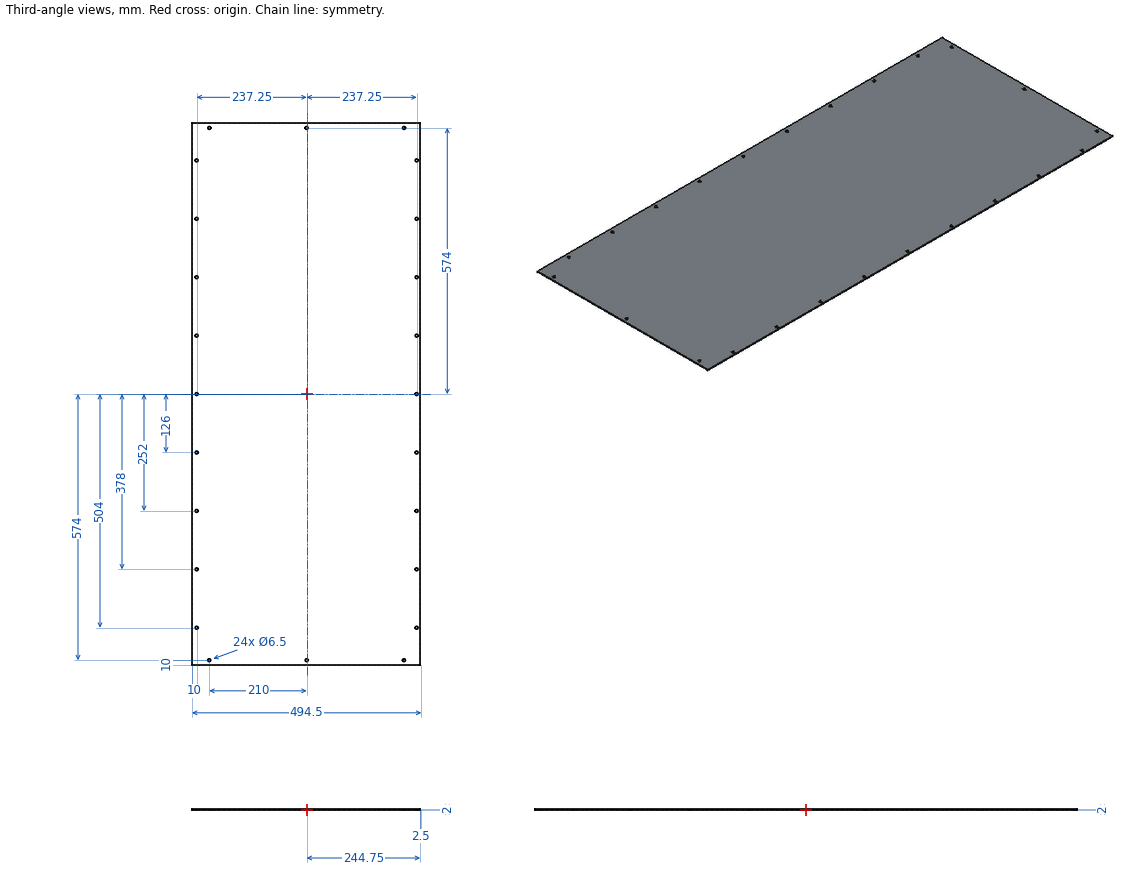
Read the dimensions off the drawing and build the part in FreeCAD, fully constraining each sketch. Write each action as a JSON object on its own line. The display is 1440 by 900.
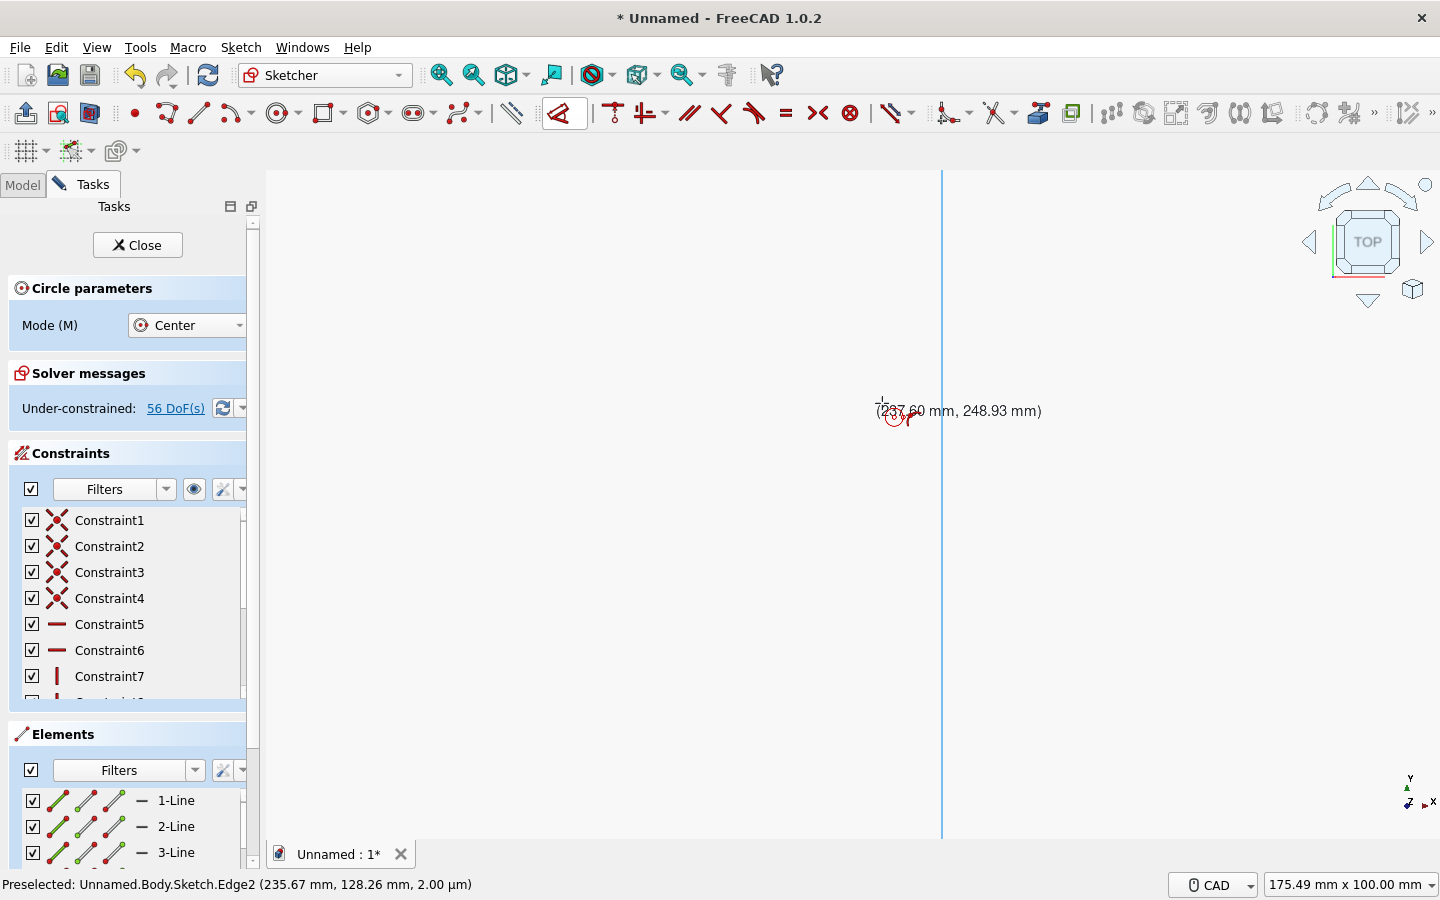
{"action": "scroll", "coordinate": [882, 403], "scroll_direction": "down", "scroll_amount": 15}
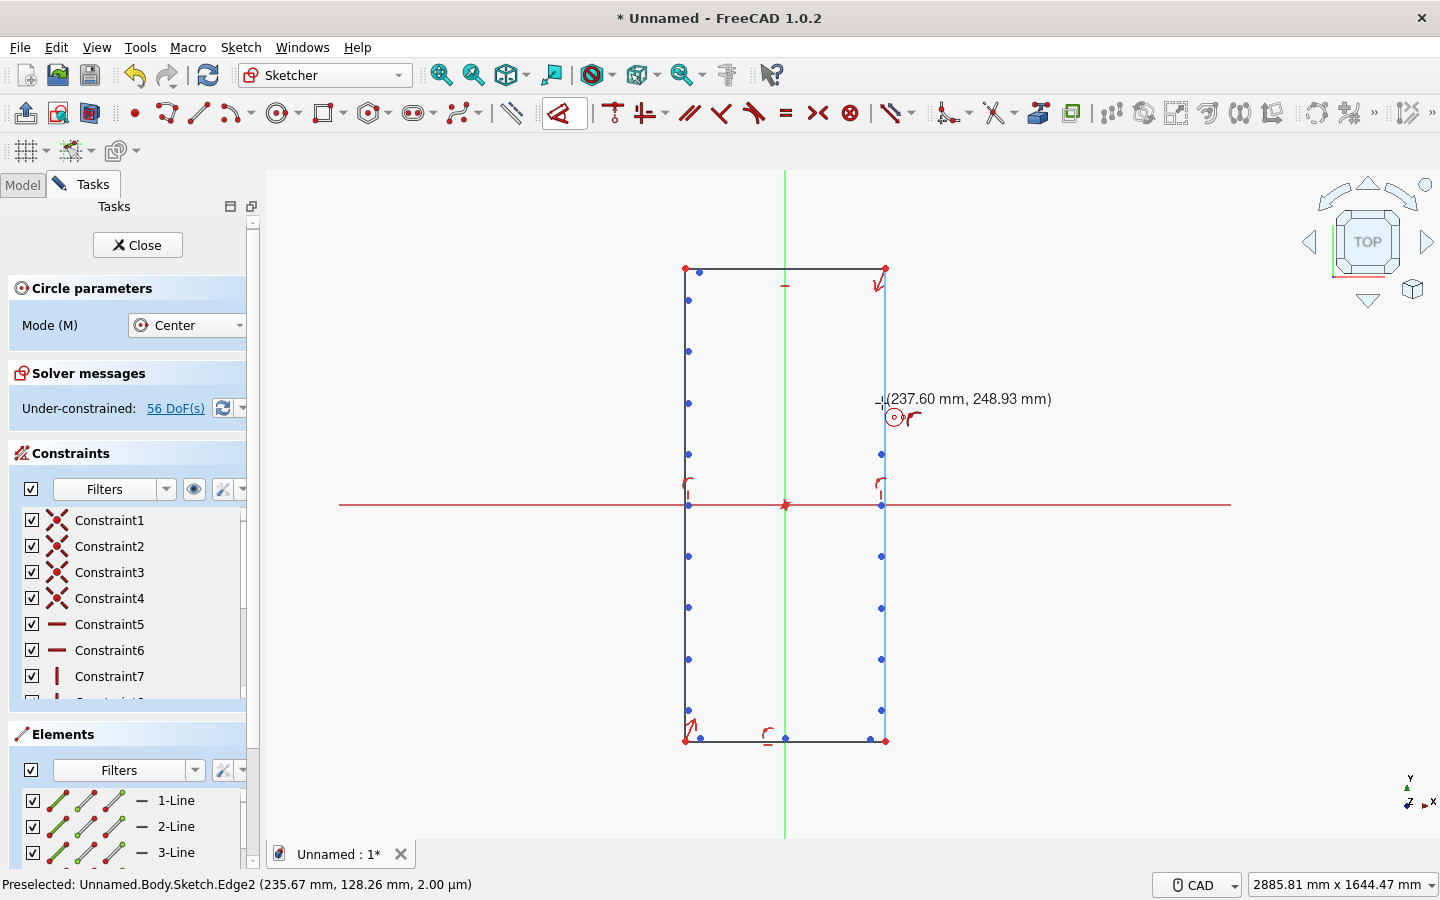
{"action": "scroll", "coordinate": [882, 403], "scroll_direction": "up", "scroll_amount": 7}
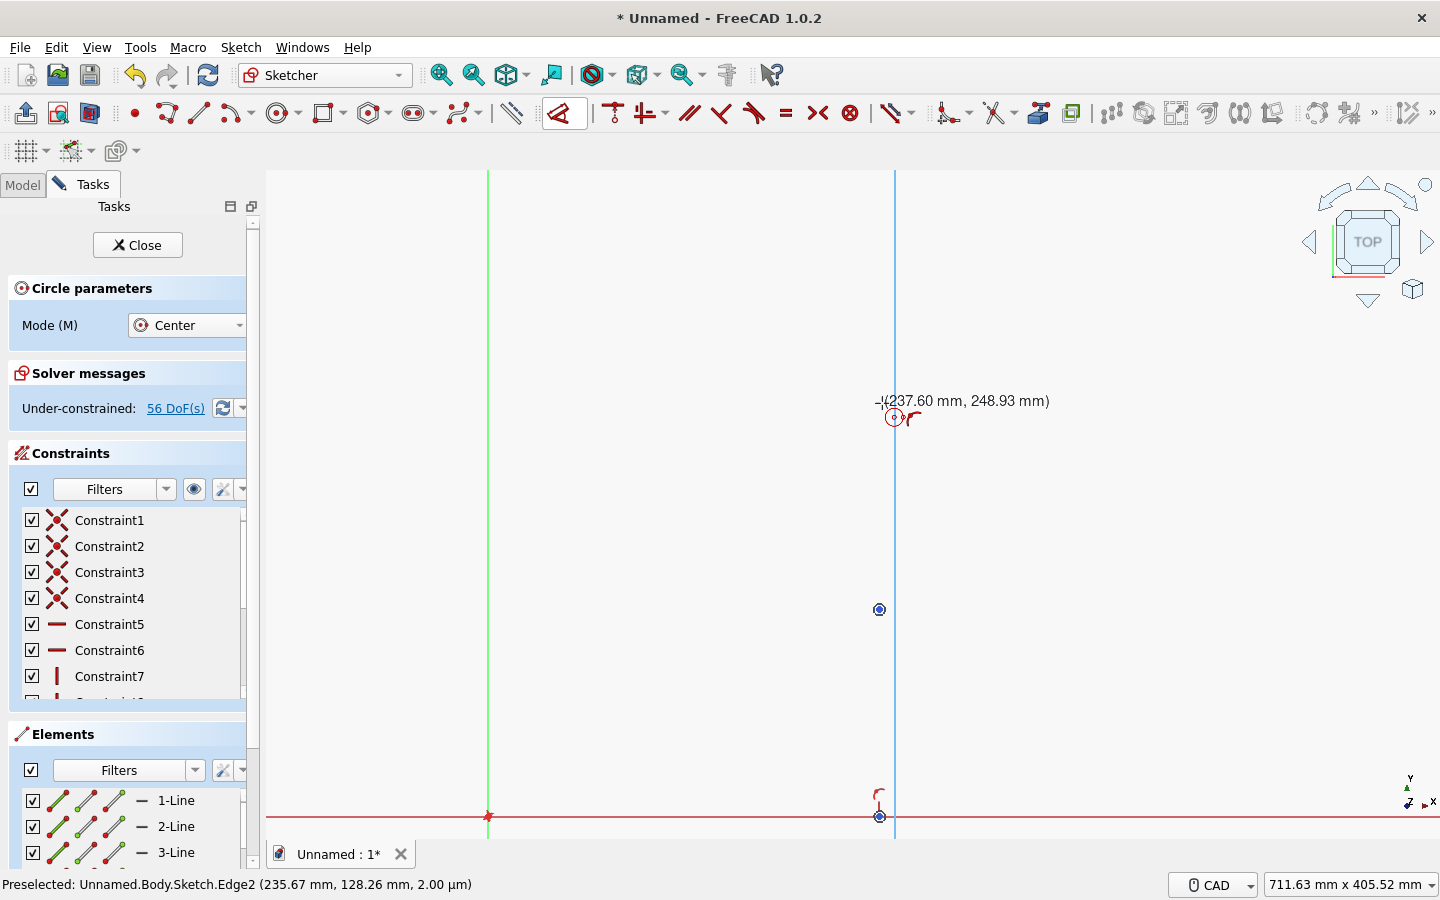
{"action": "left_click", "coordinate": [880, 401]}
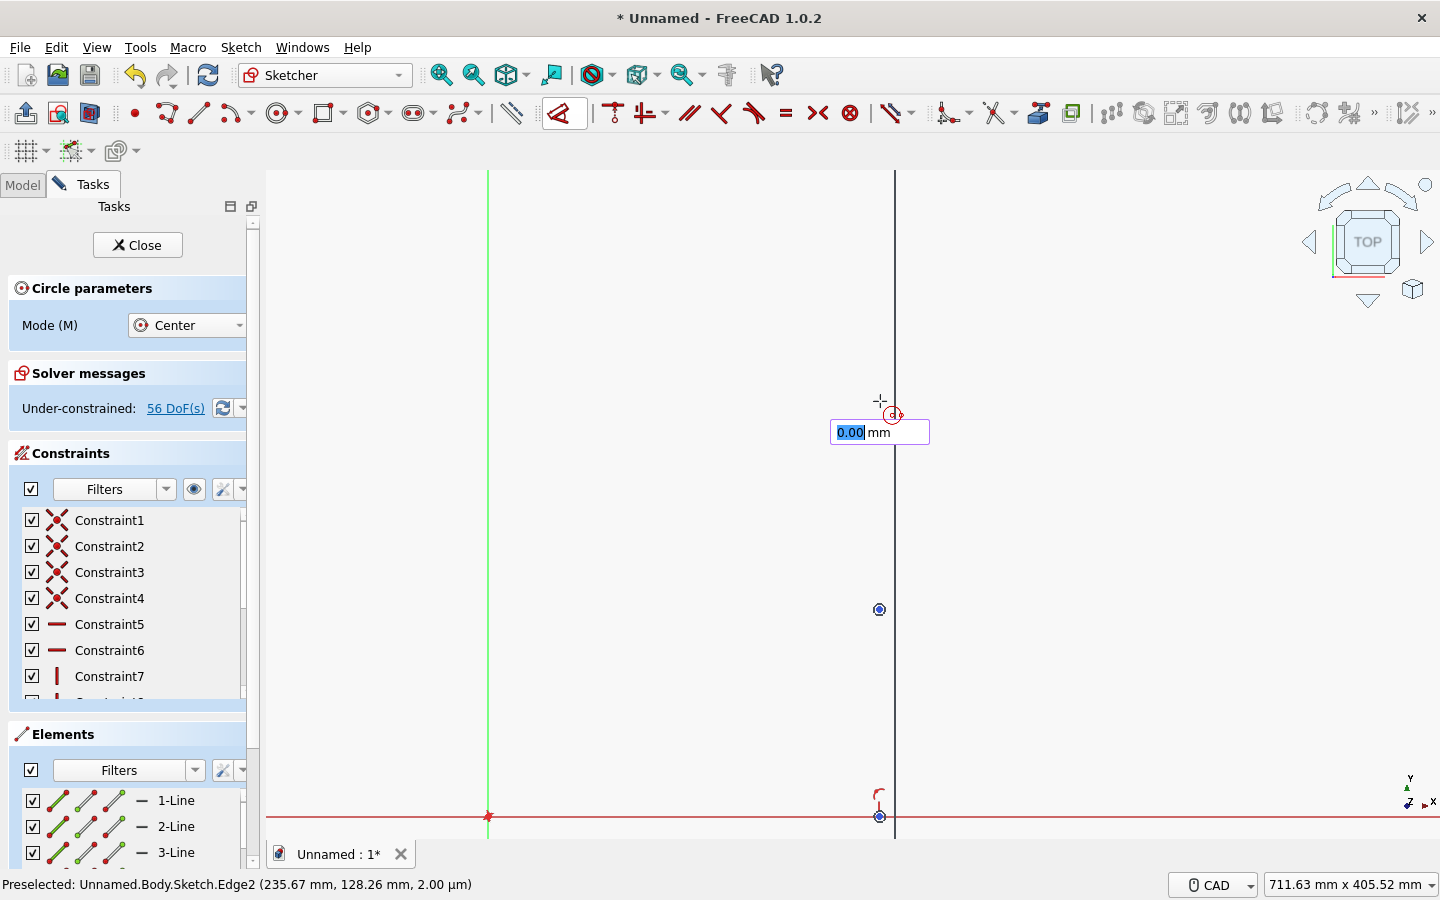
{"action": "scroll", "coordinate": [876, 397], "scroll_direction": "up", "scroll_amount": 6}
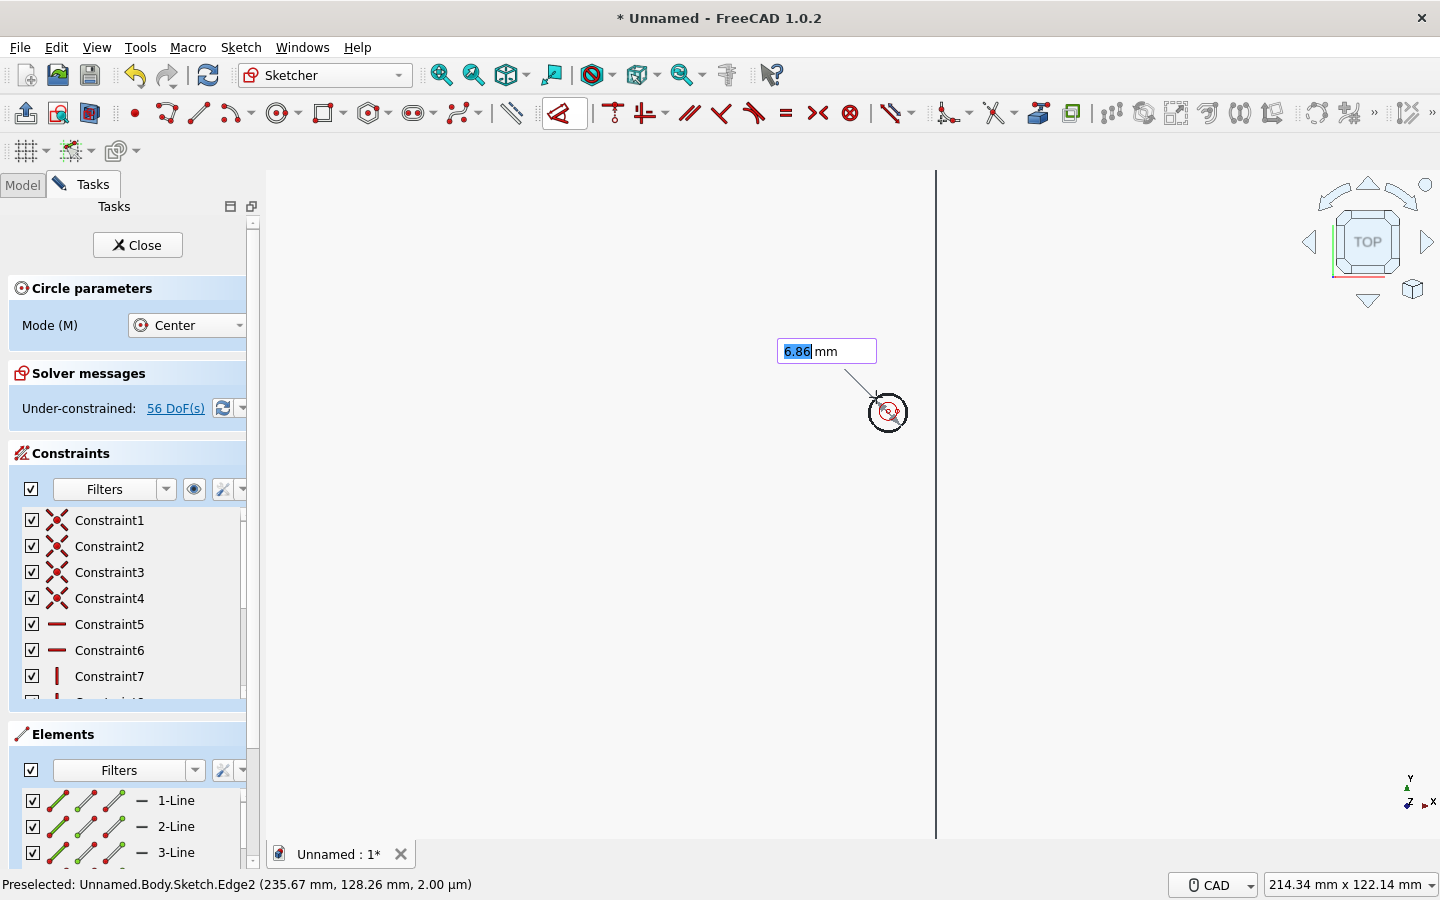
{"action": "left_click", "coordinate": [875, 397]}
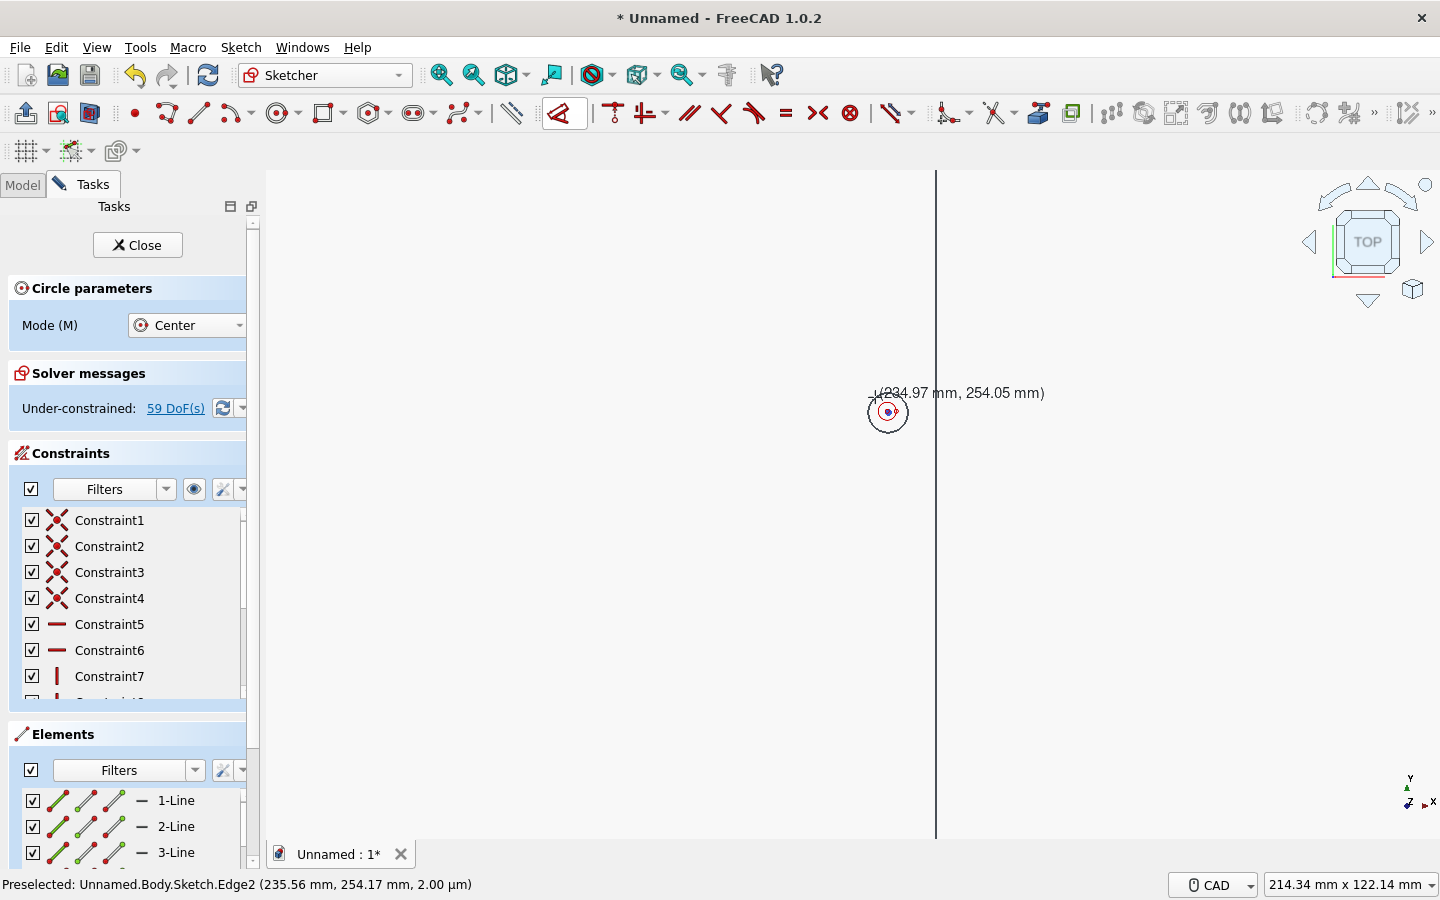
{"action": "scroll", "coordinate": [880, 401], "scroll_direction": "down", "scroll_amount": 13}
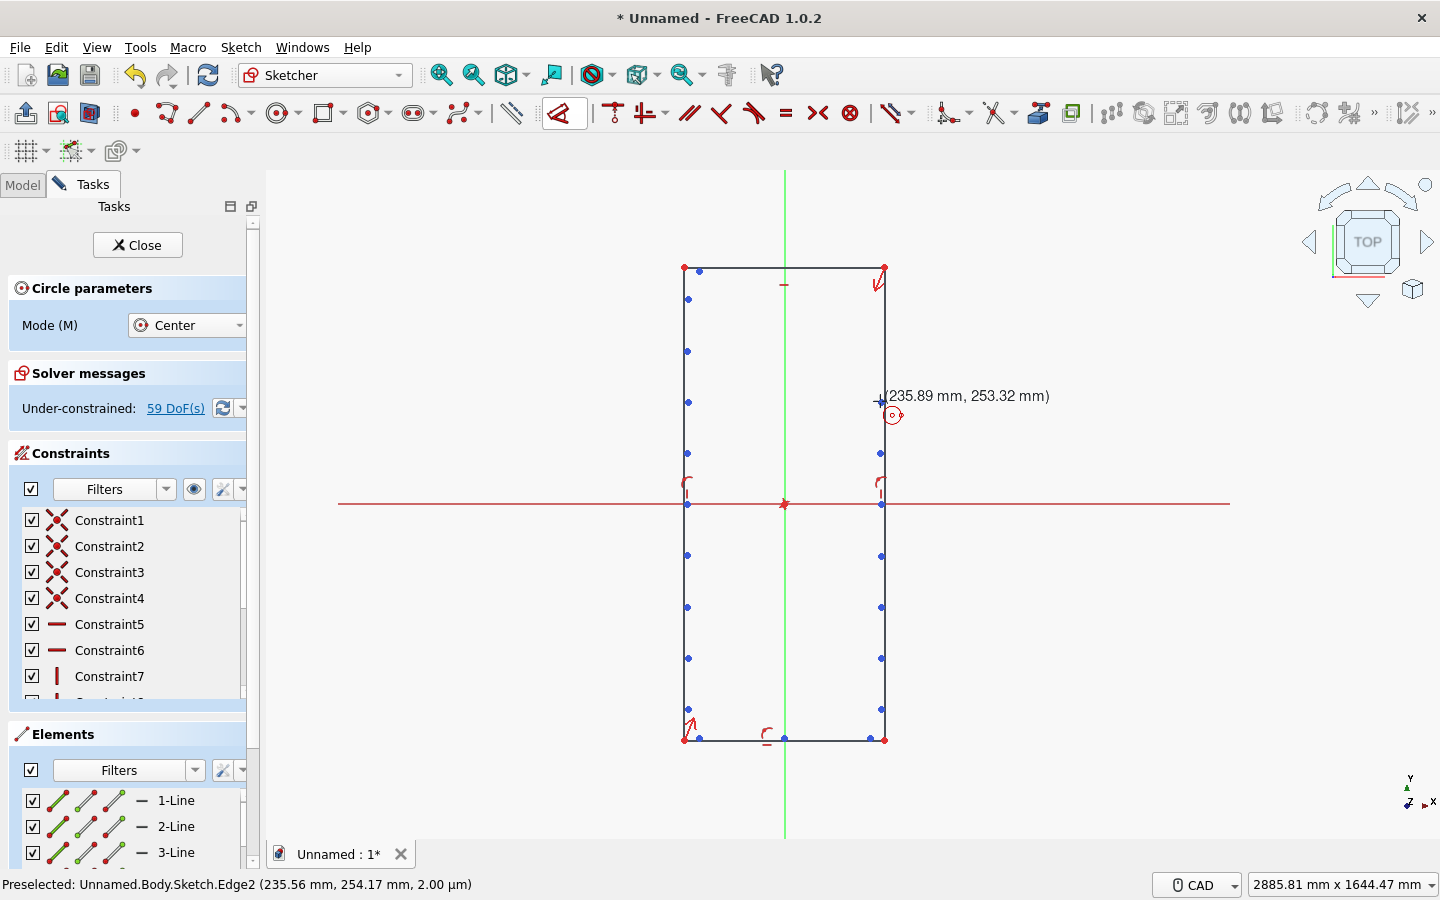
{"action": "scroll", "coordinate": [785, 271], "scroll_direction": "up", "scroll_amount": 15}